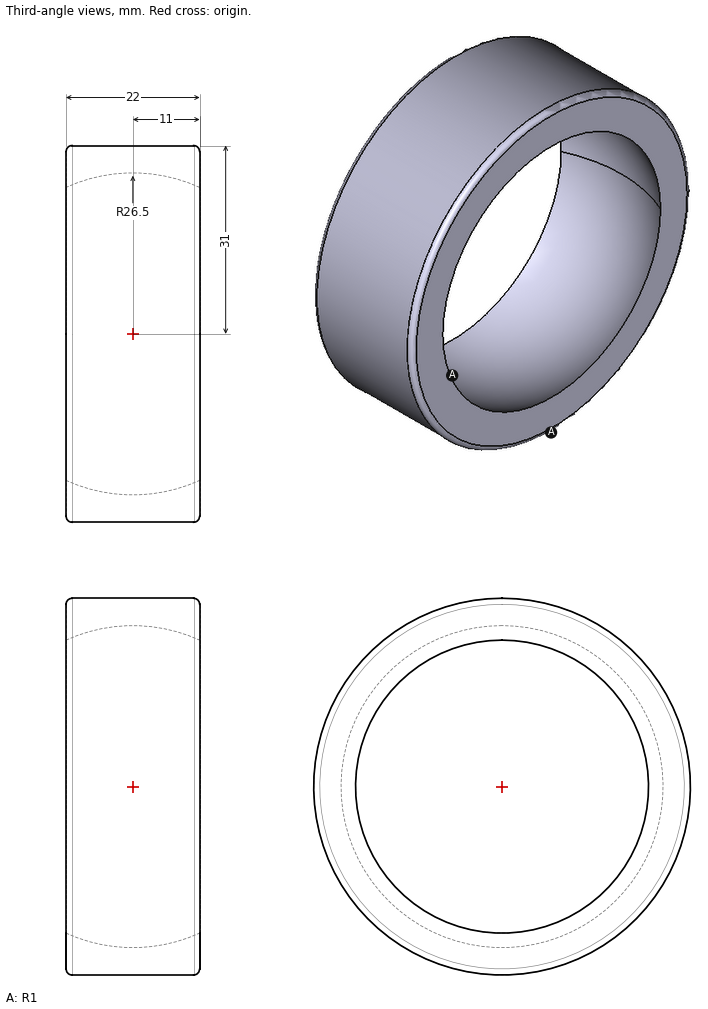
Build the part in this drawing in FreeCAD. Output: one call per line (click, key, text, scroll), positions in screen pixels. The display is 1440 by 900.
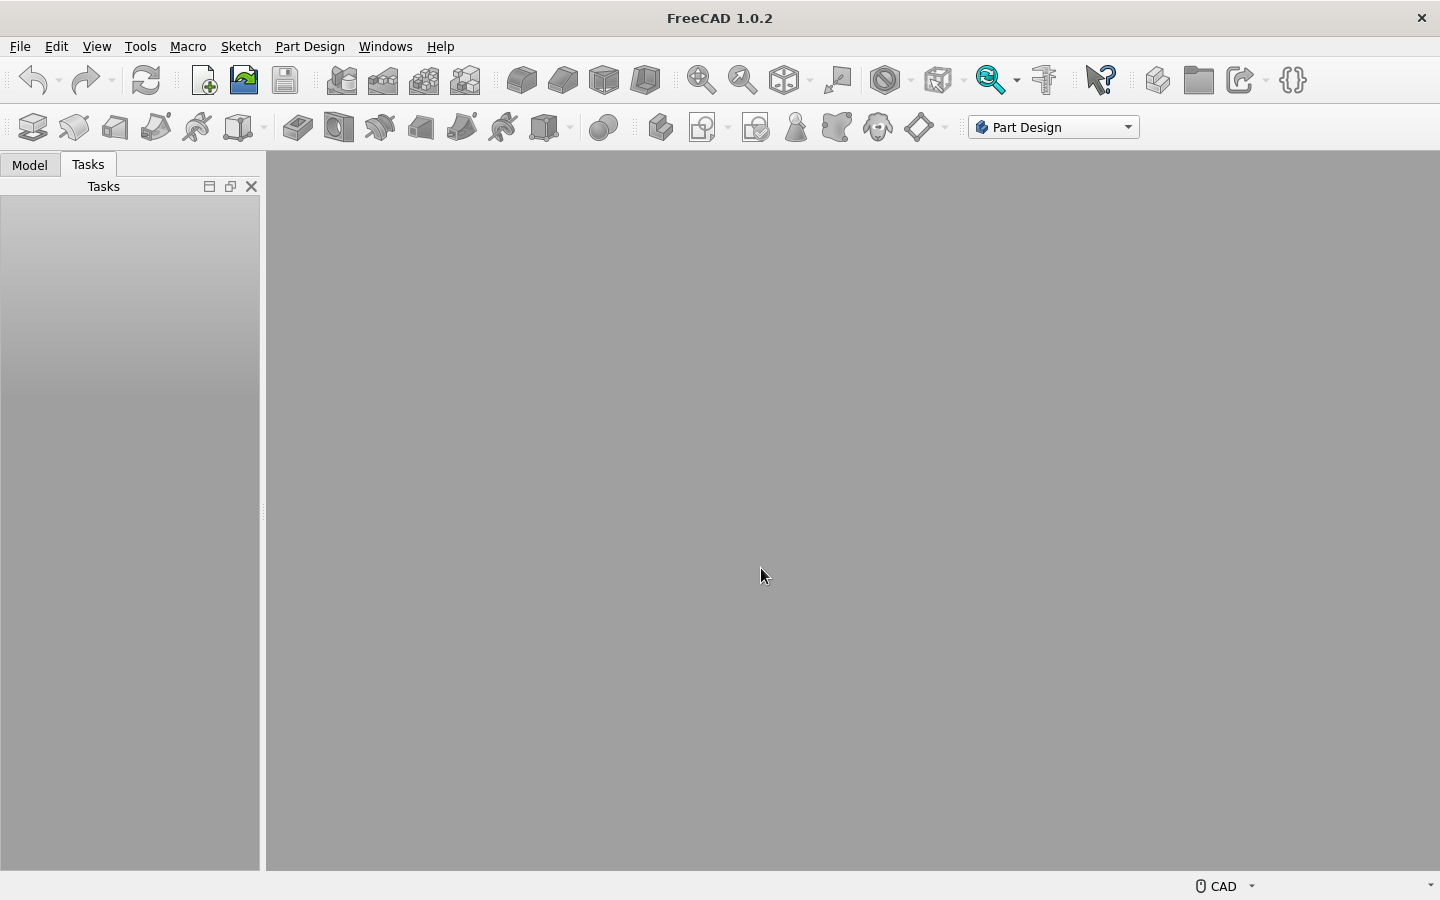
click(203, 80)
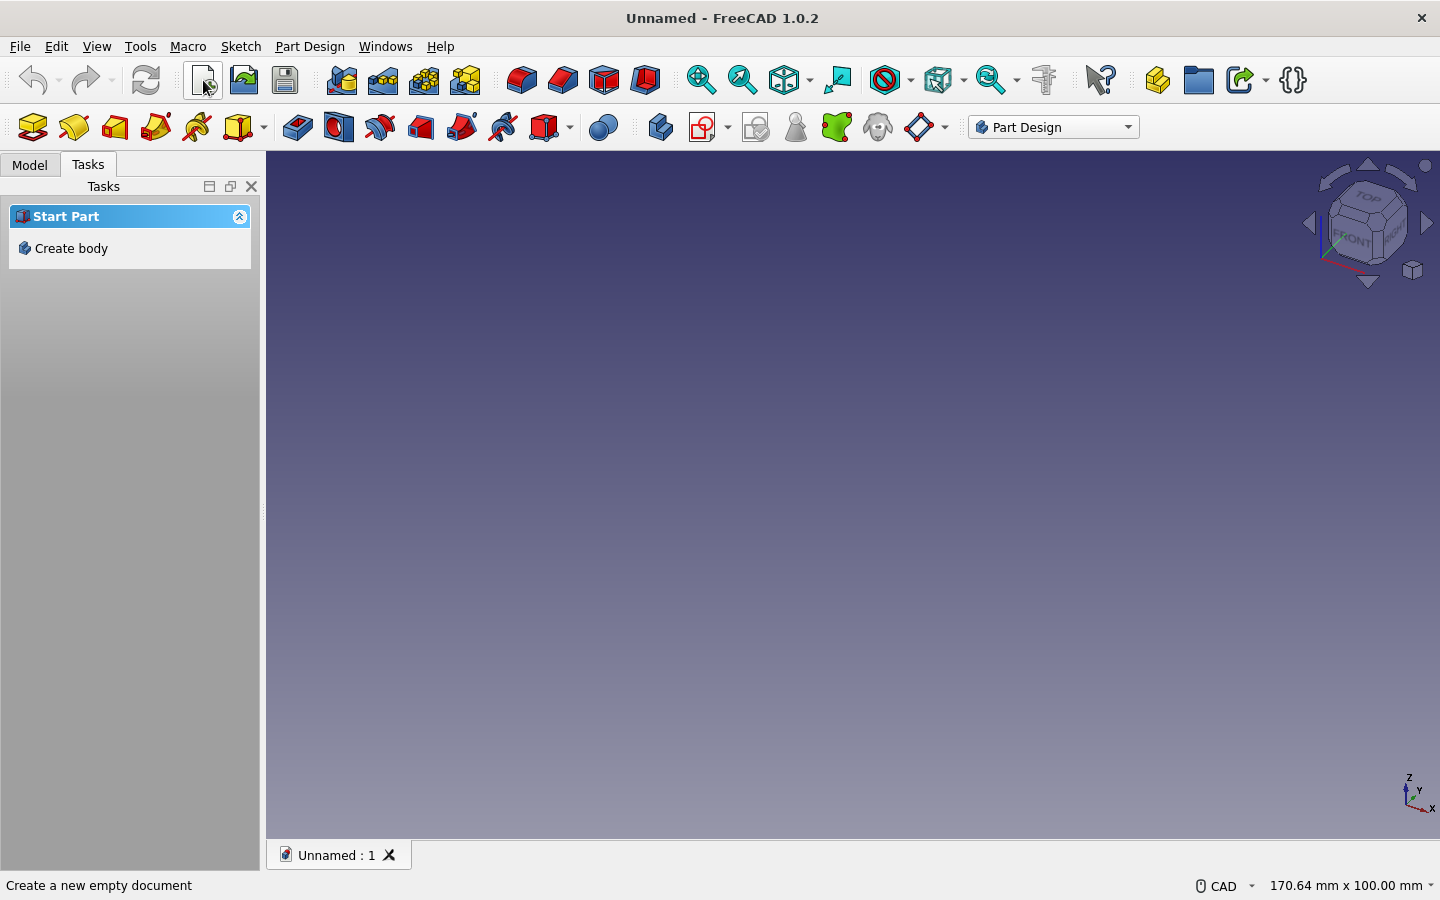
click(702, 128)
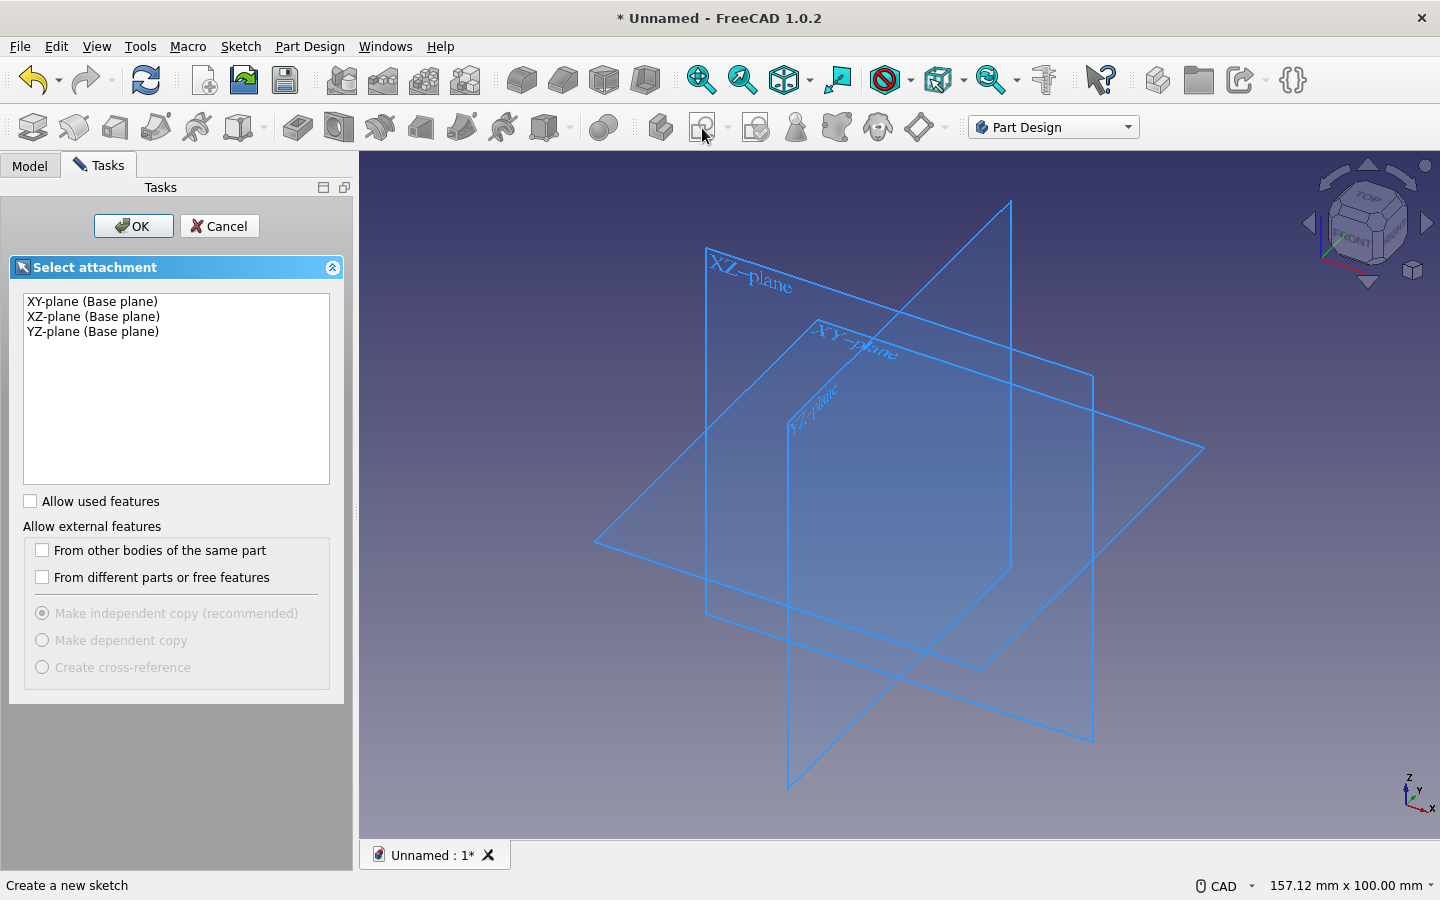
click(84, 302)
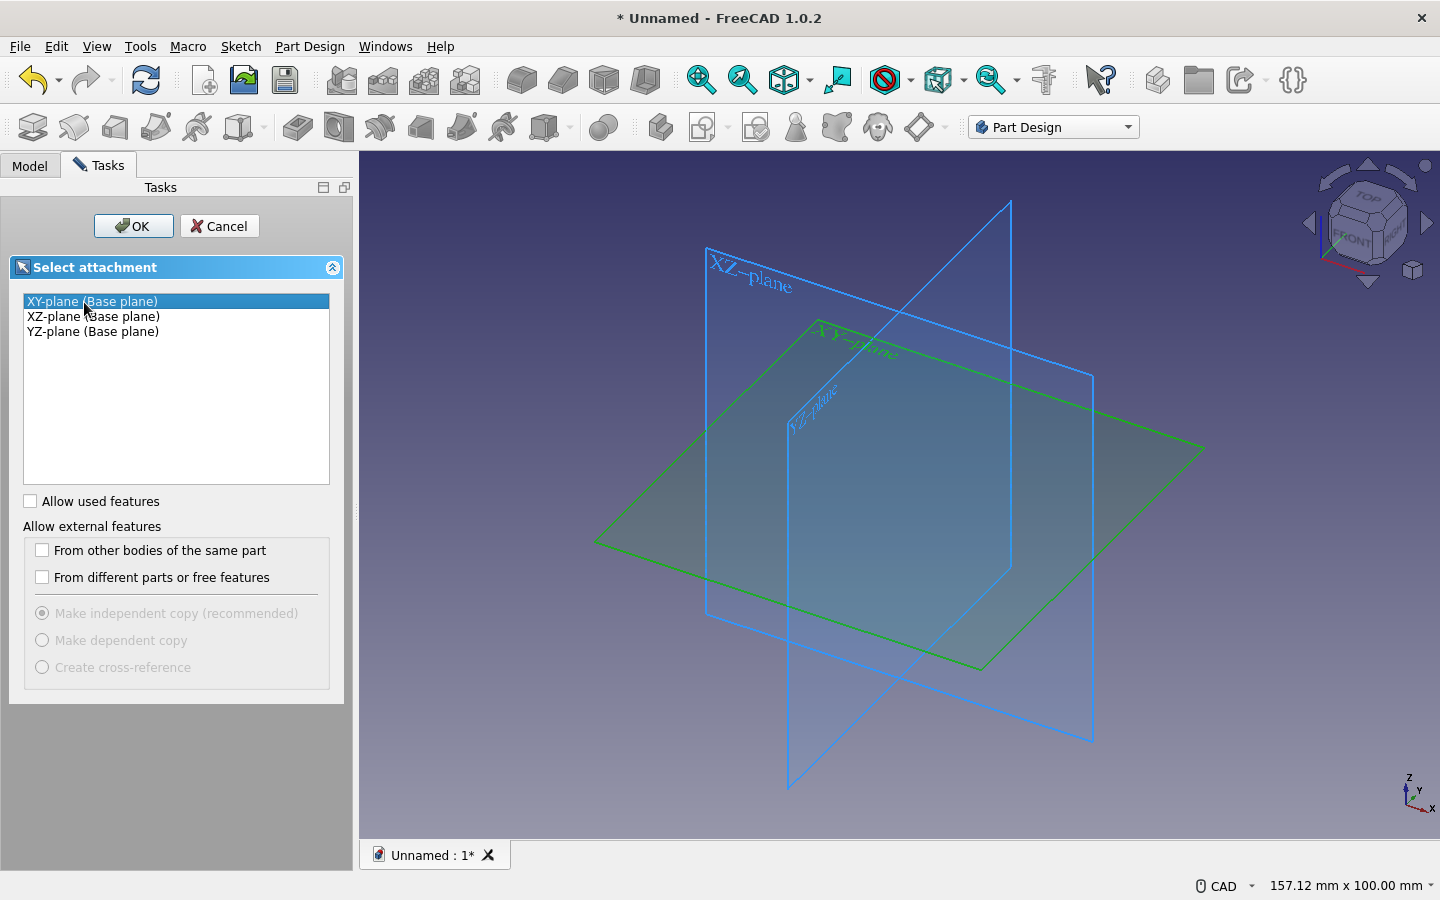
click(134, 226)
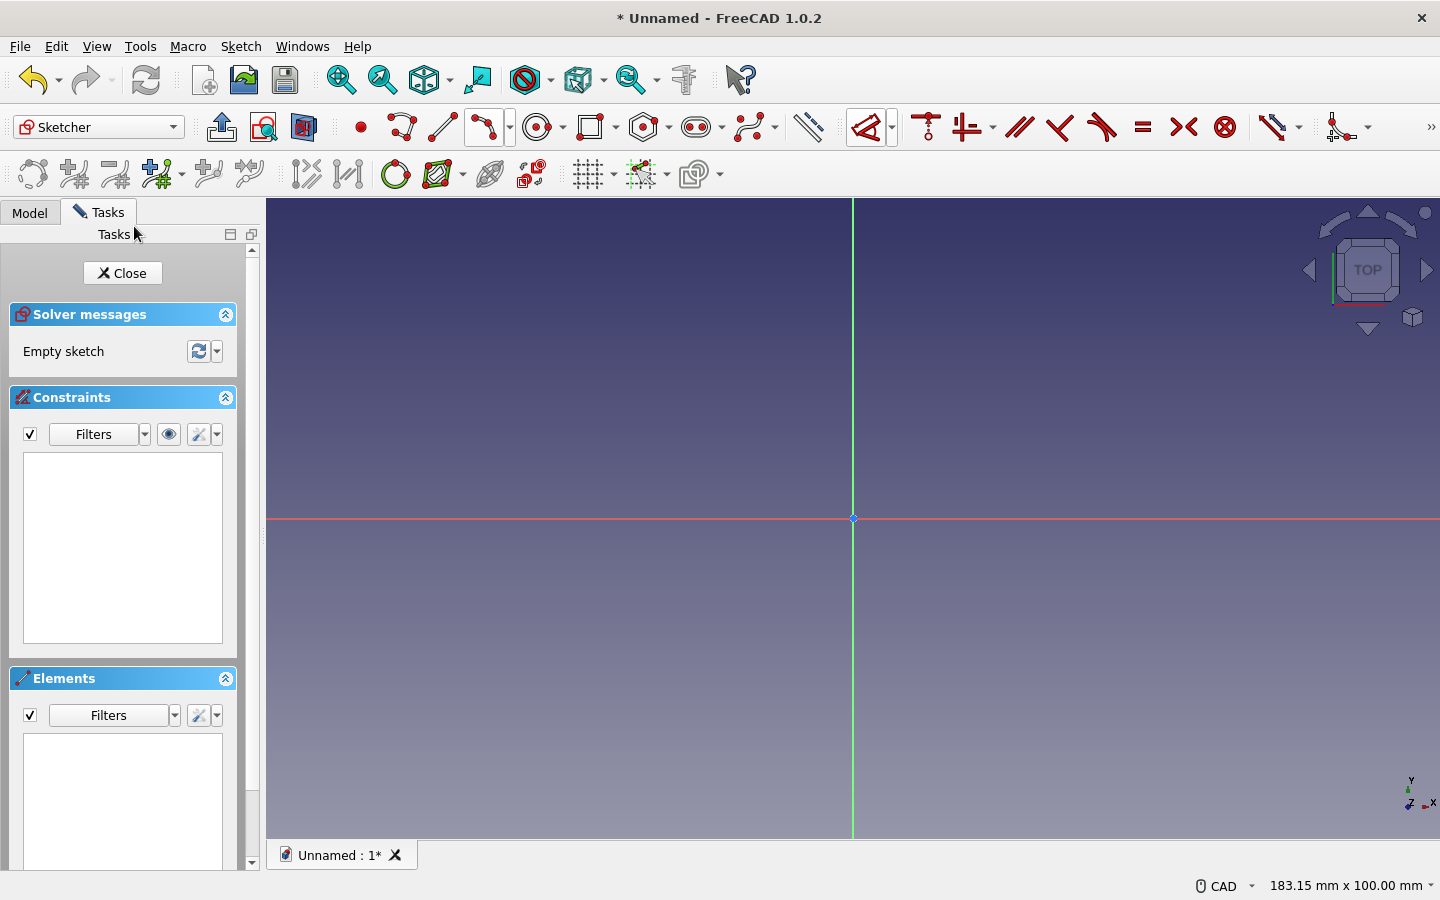
scroll(909, 338, up, 4)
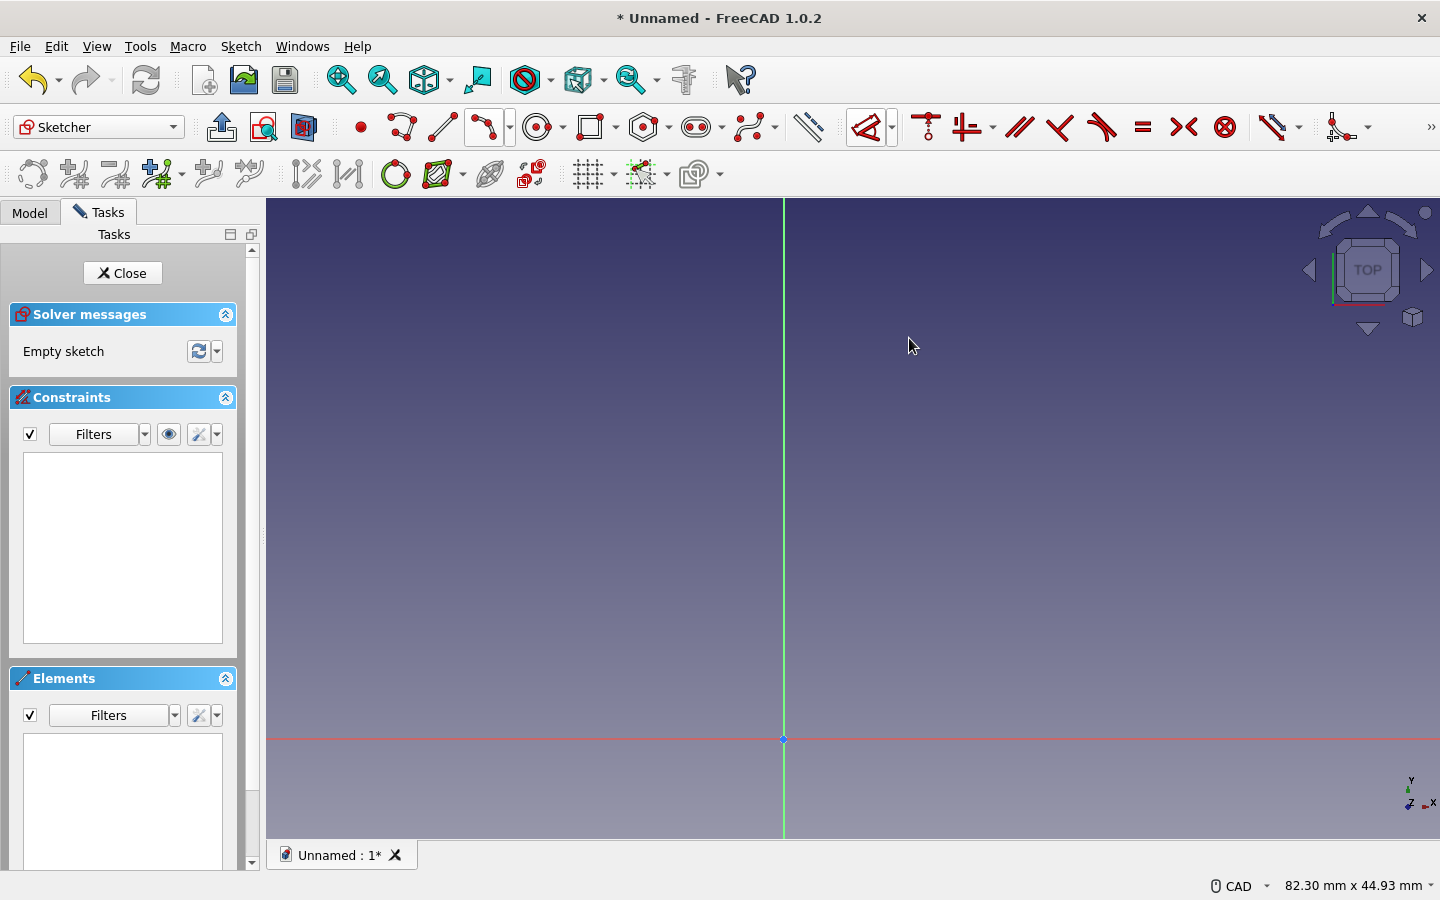
click(402, 128)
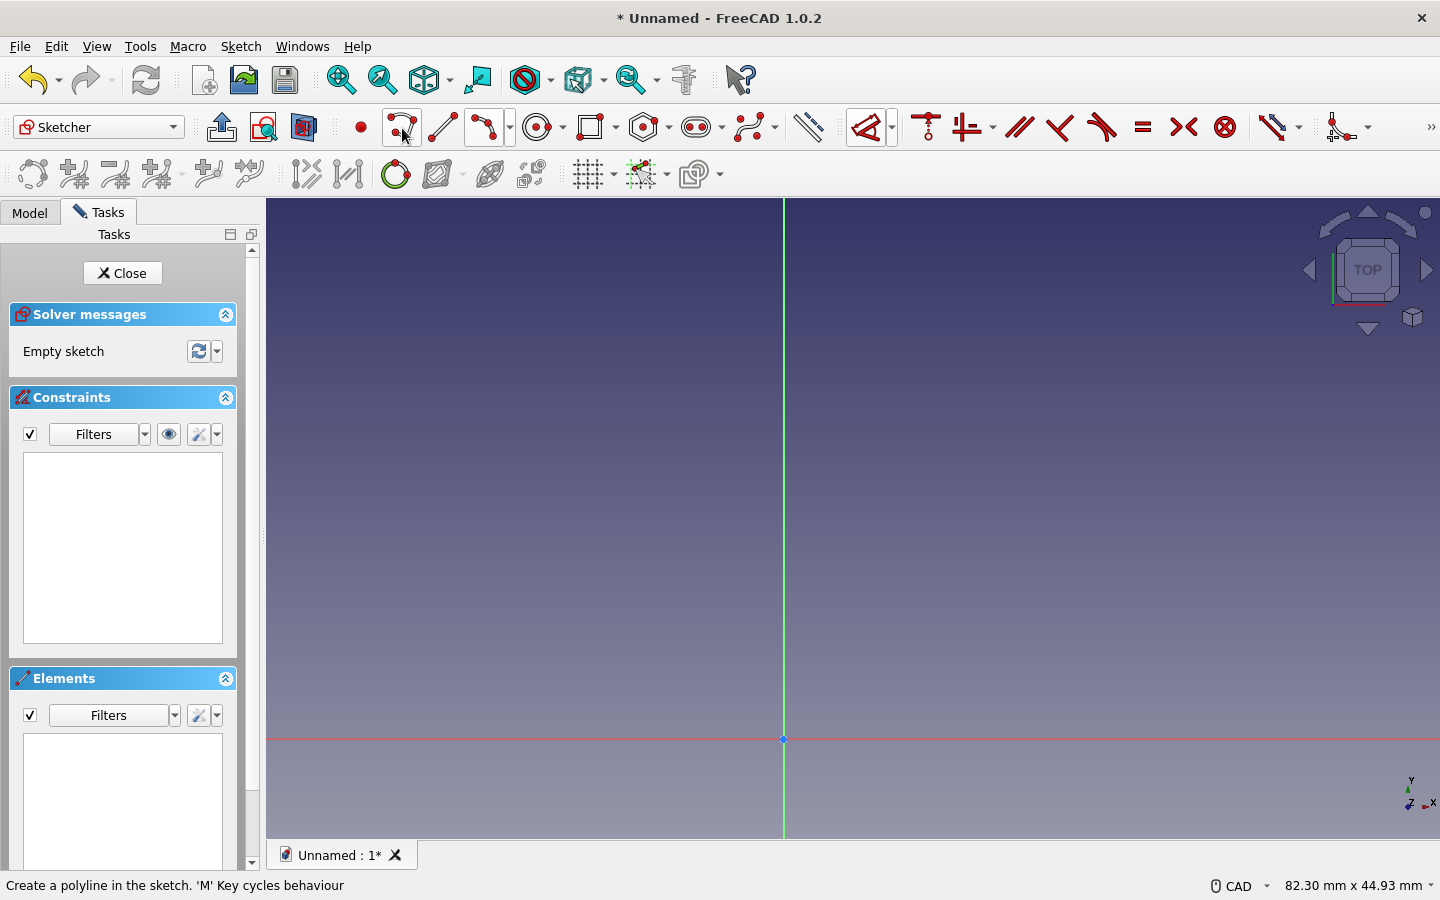
click(941, 396)
click(941, 297)
click(627, 297)
click(627, 396)
right_click(627, 396)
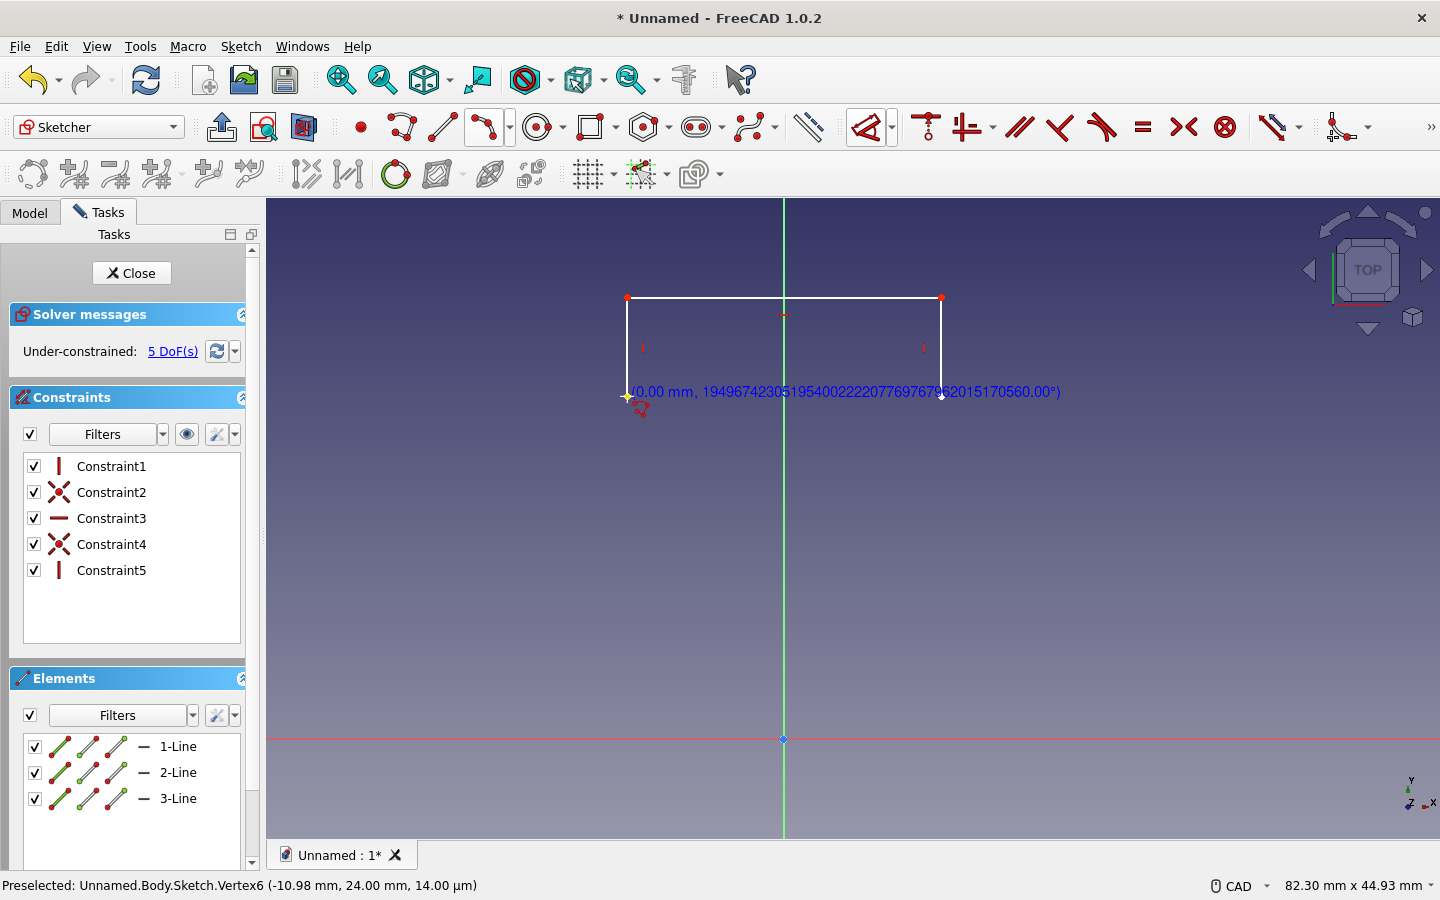
click(484, 128)